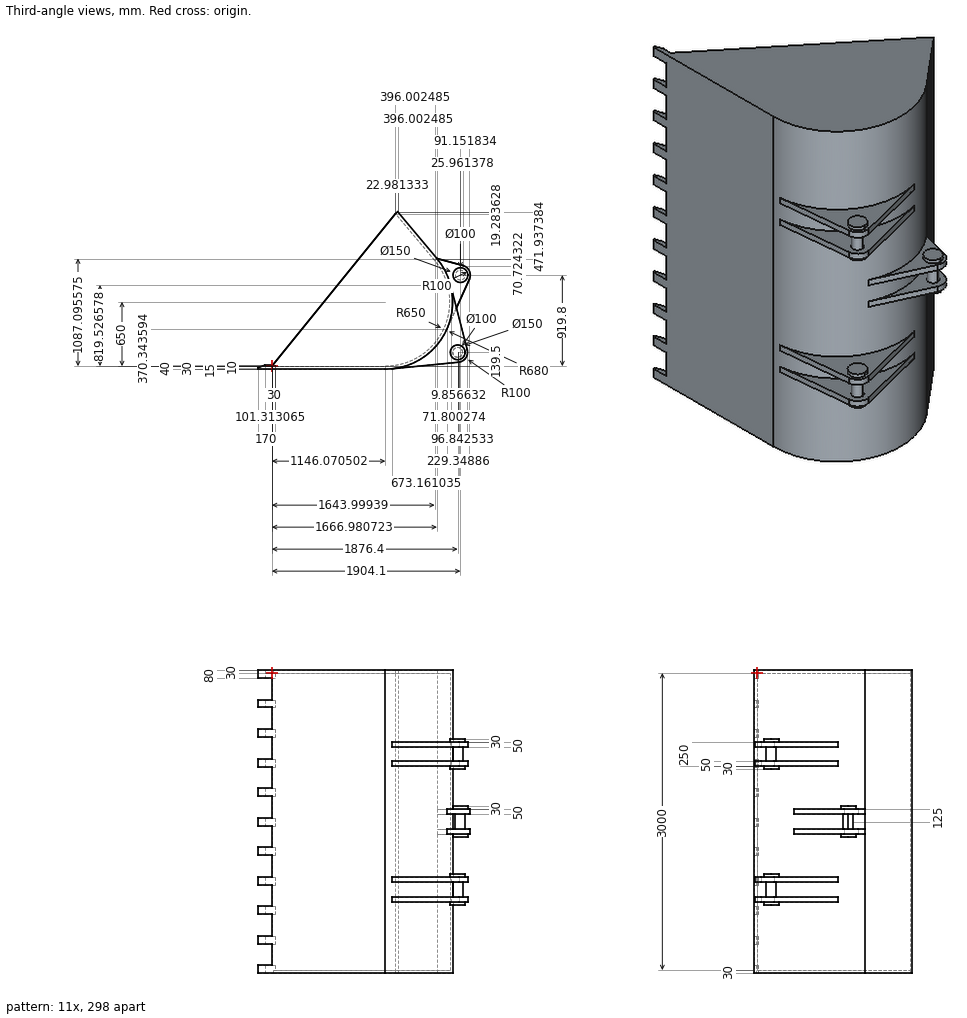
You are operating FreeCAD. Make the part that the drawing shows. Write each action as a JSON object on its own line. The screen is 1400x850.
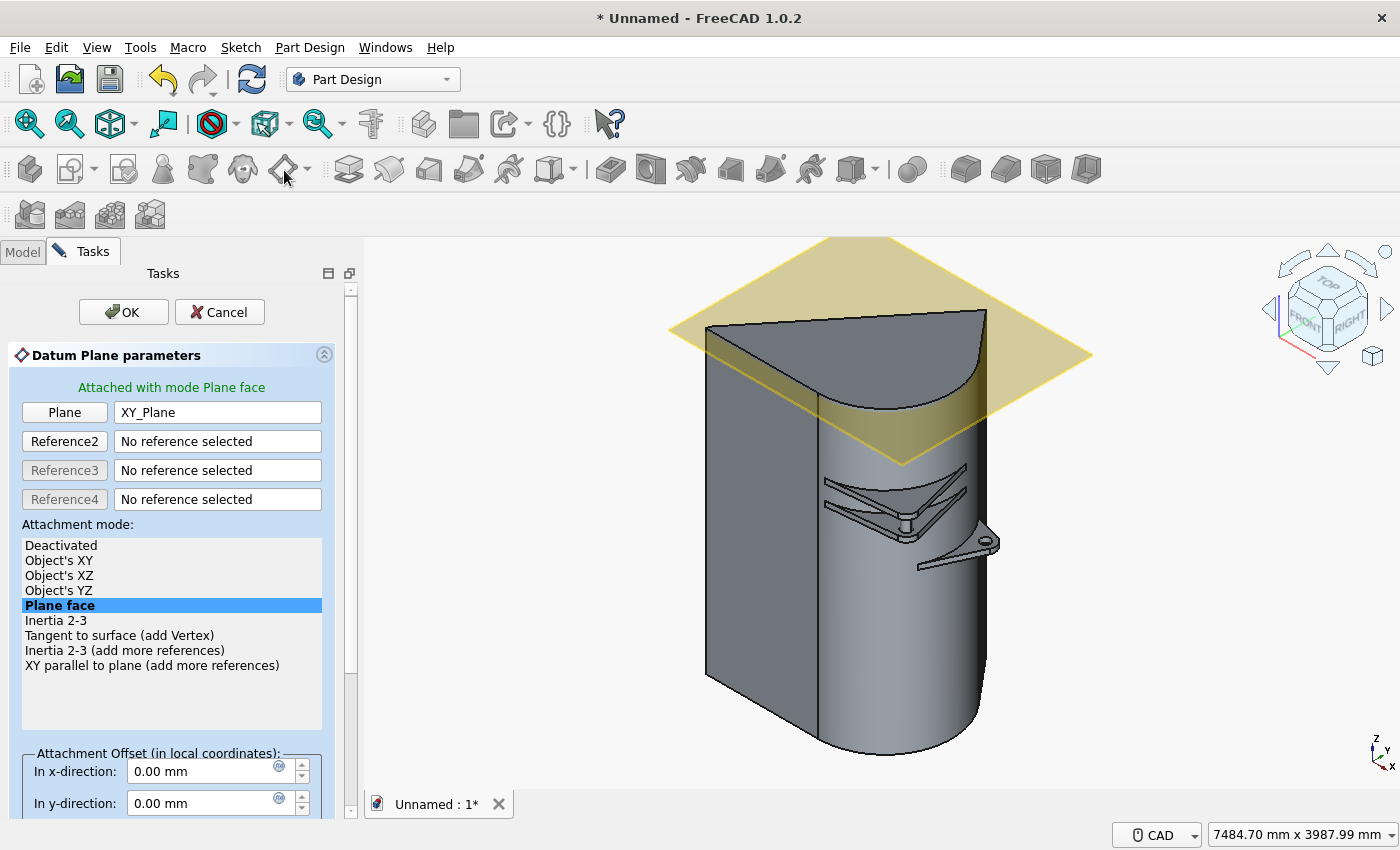
{"action": "scroll", "coordinate": [351, 550], "scroll_direction": "down", "scroll_amount": 2}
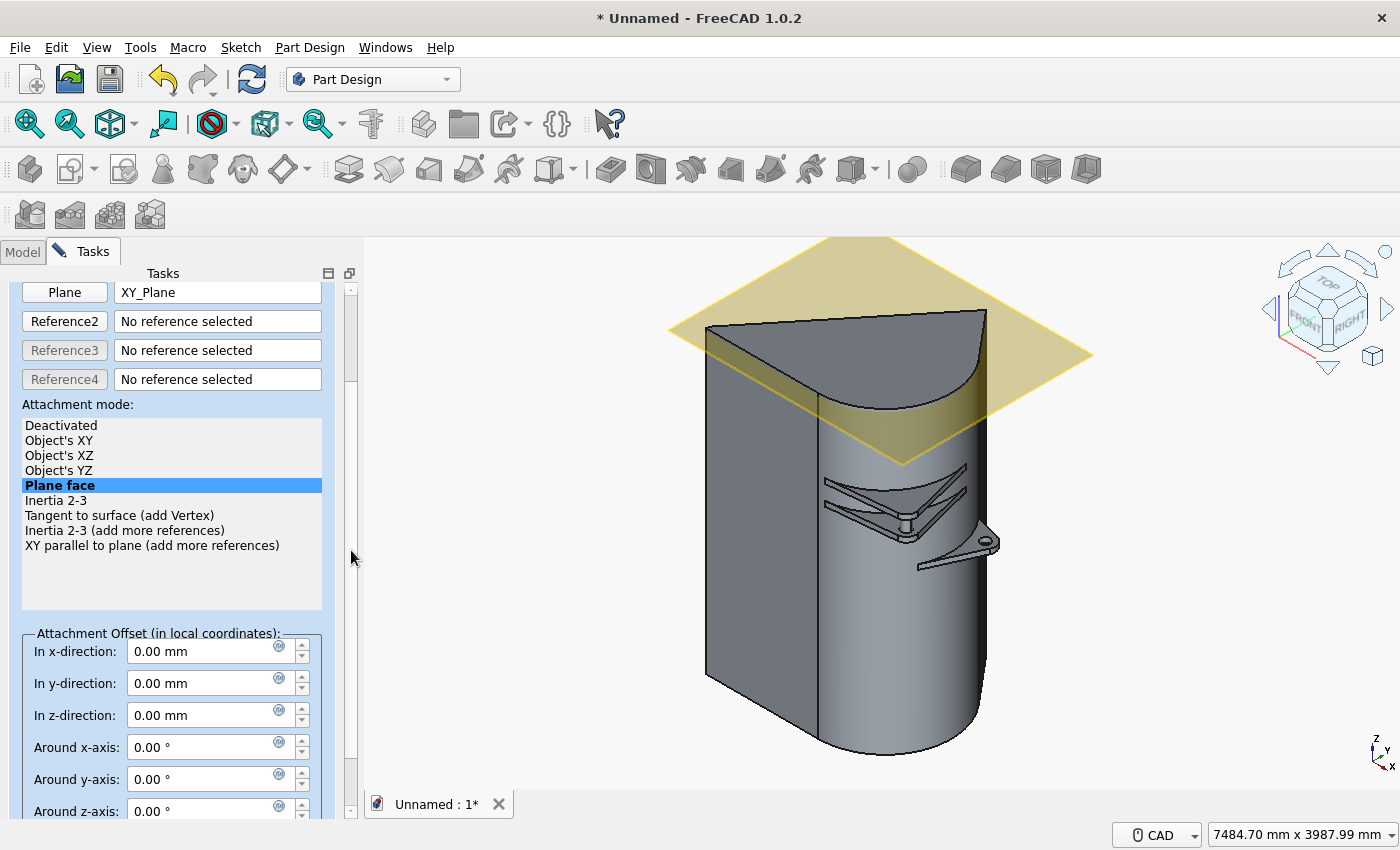
{"action": "triple_click", "coordinate": [210, 715]}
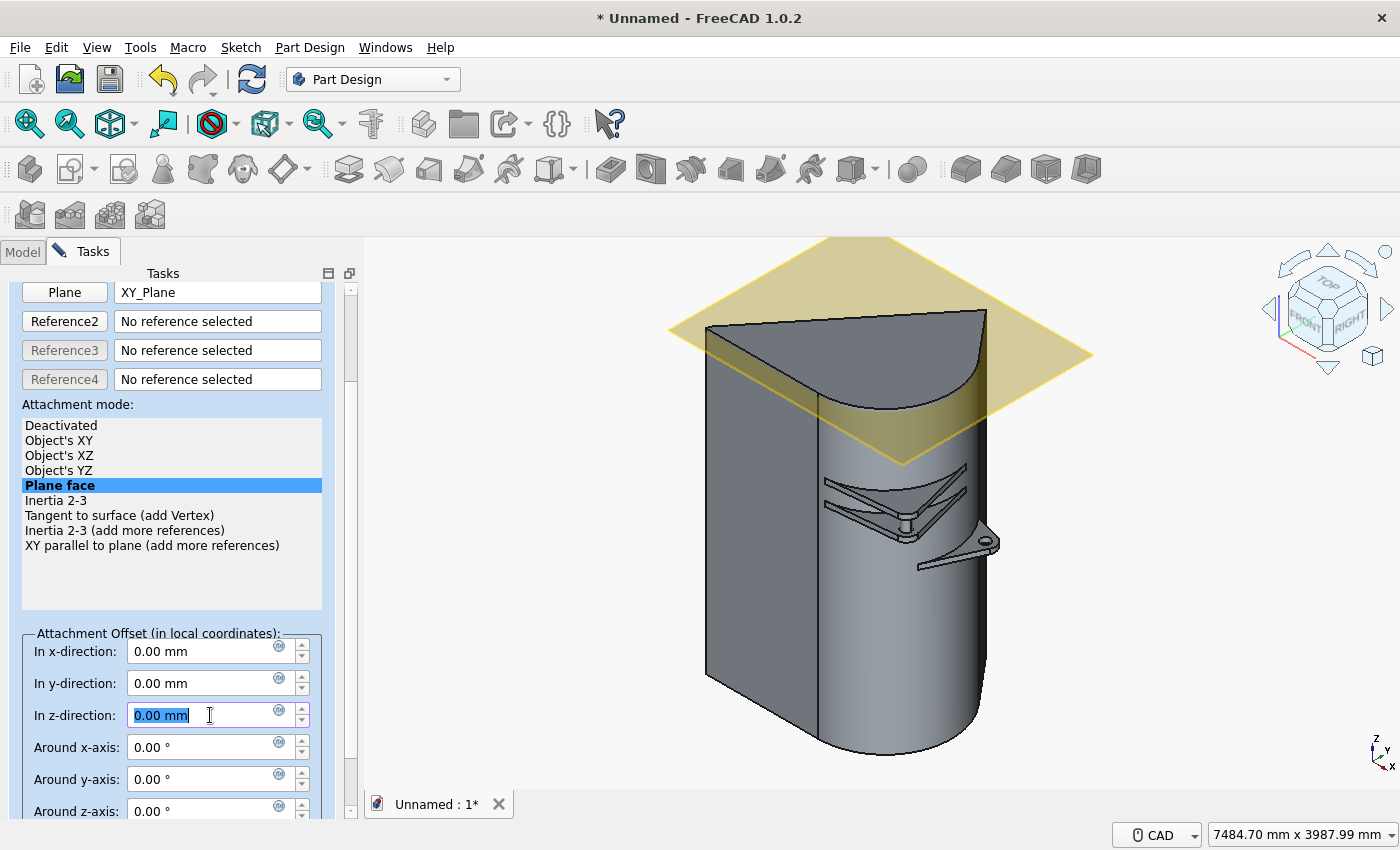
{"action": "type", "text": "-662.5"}
{"action": "key", "text": "Tab"}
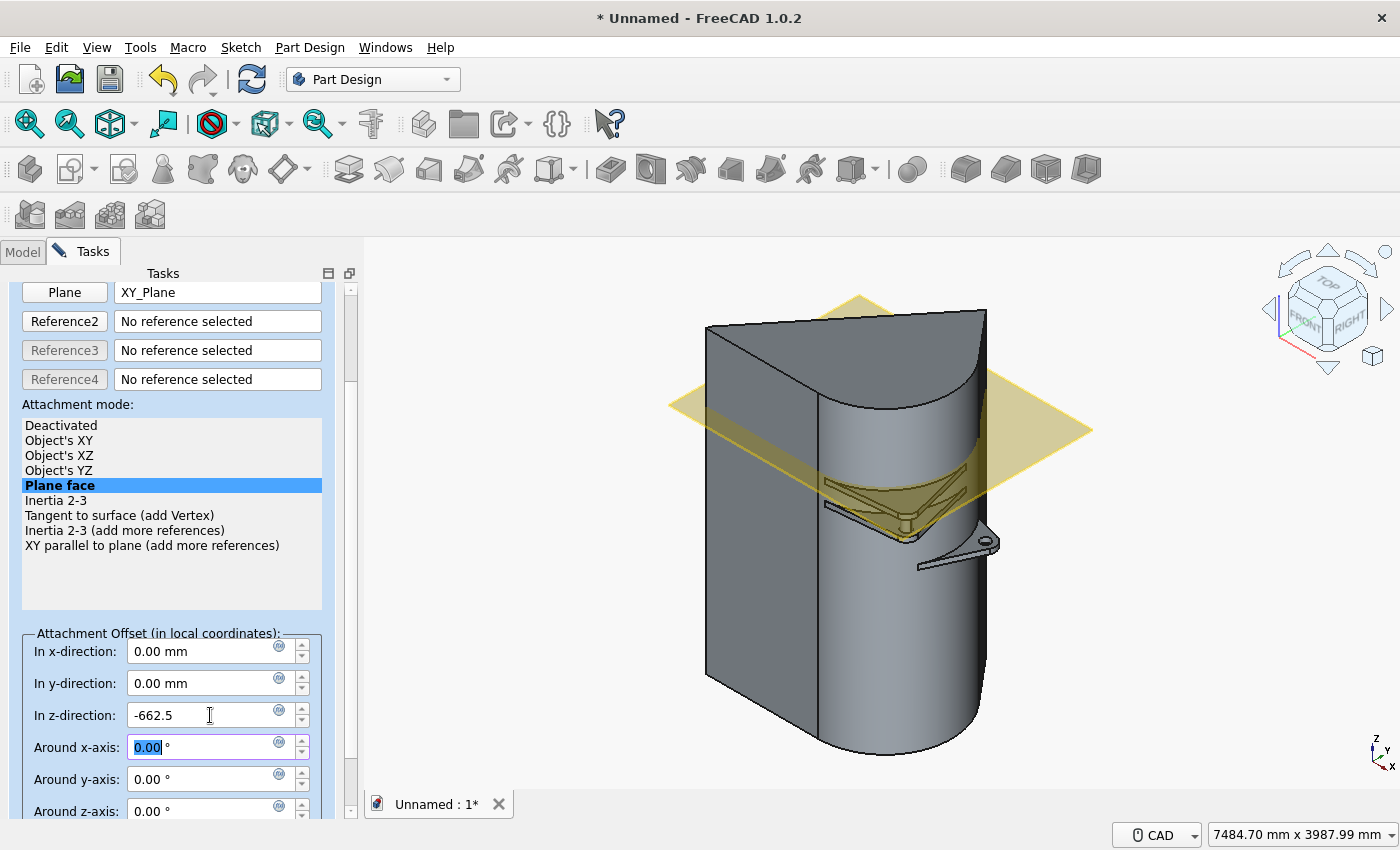
{"action": "scroll", "coordinate": [351, 550], "scroll_direction": "up", "scroll_amount": 3}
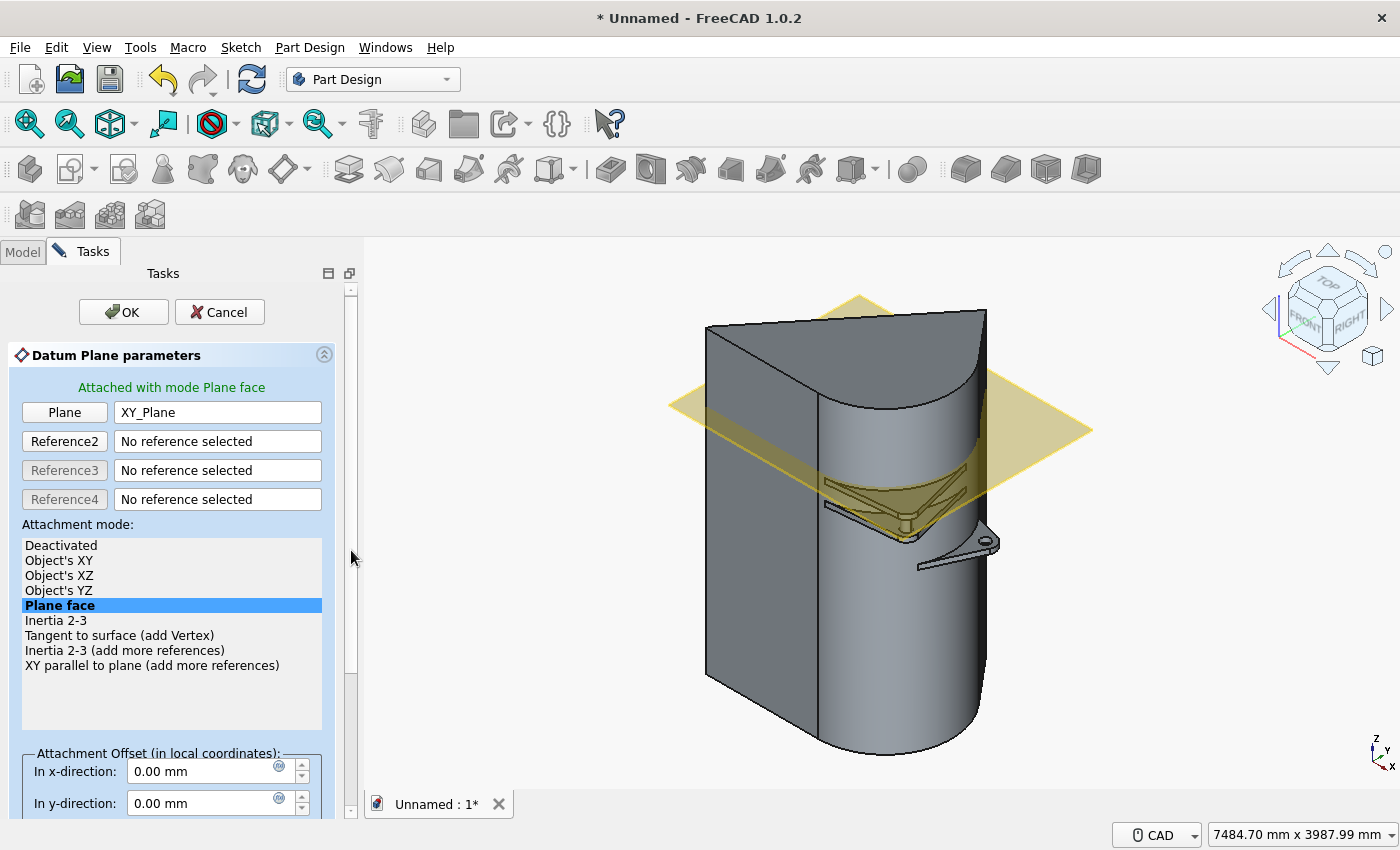
{"action": "left_click", "coordinate": [124, 312]}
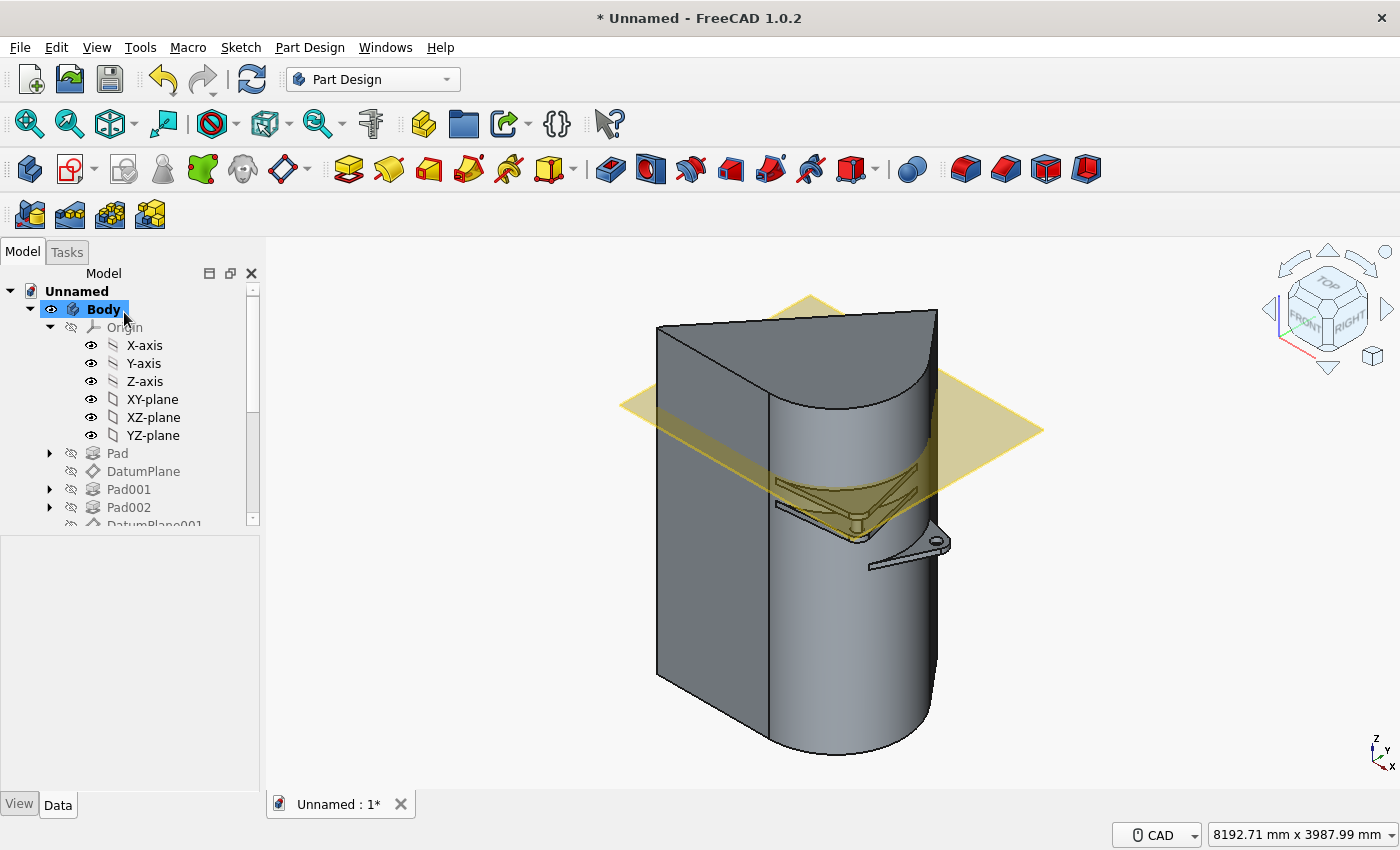
{"action": "scroll", "coordinate": [100, 413], "scroll_direction": "down", "scroll_amount": 3}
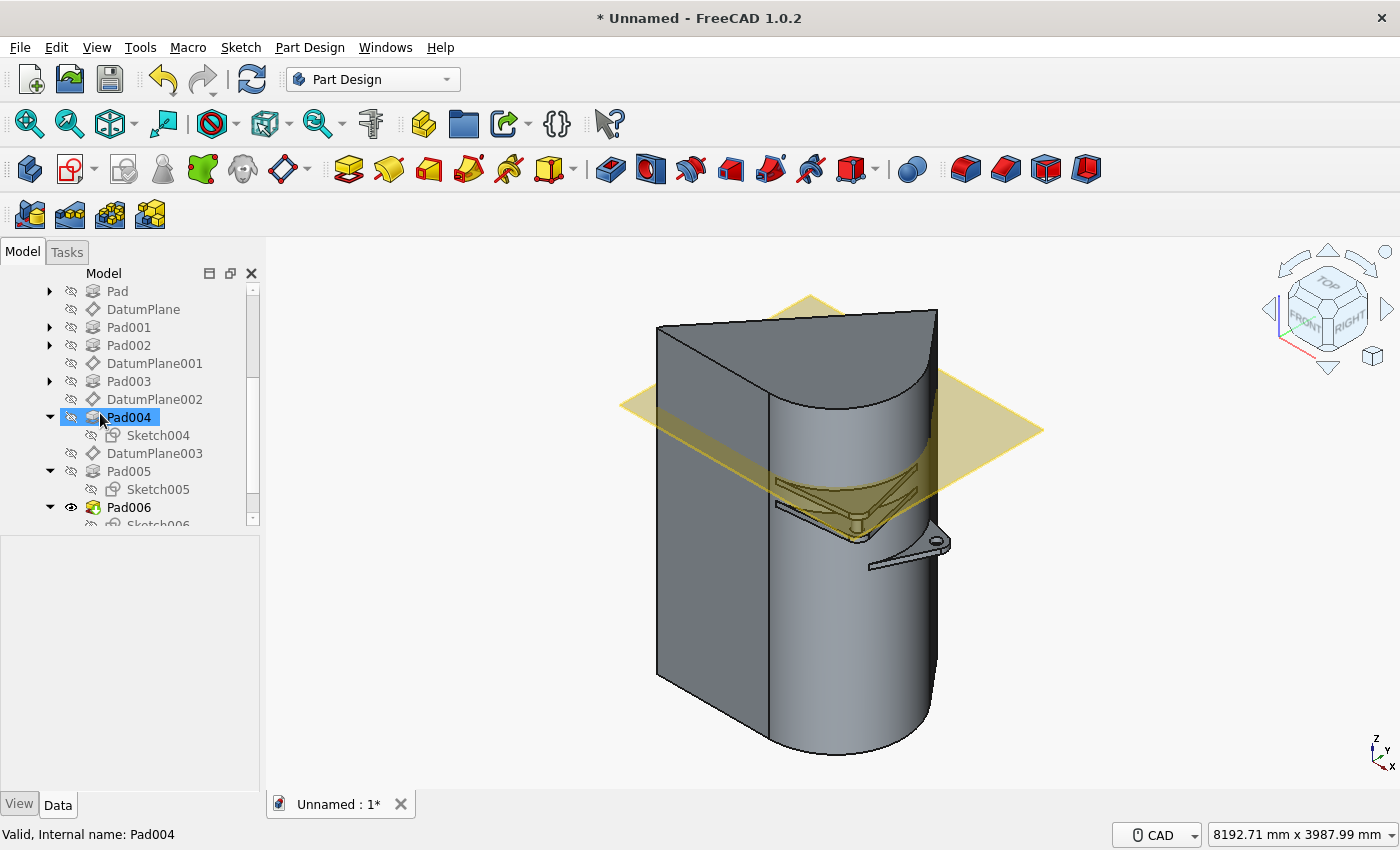
{"action": "scroll", "coordinate": [140, 413], "scroll_direction": "up", "scroll_amount": 15}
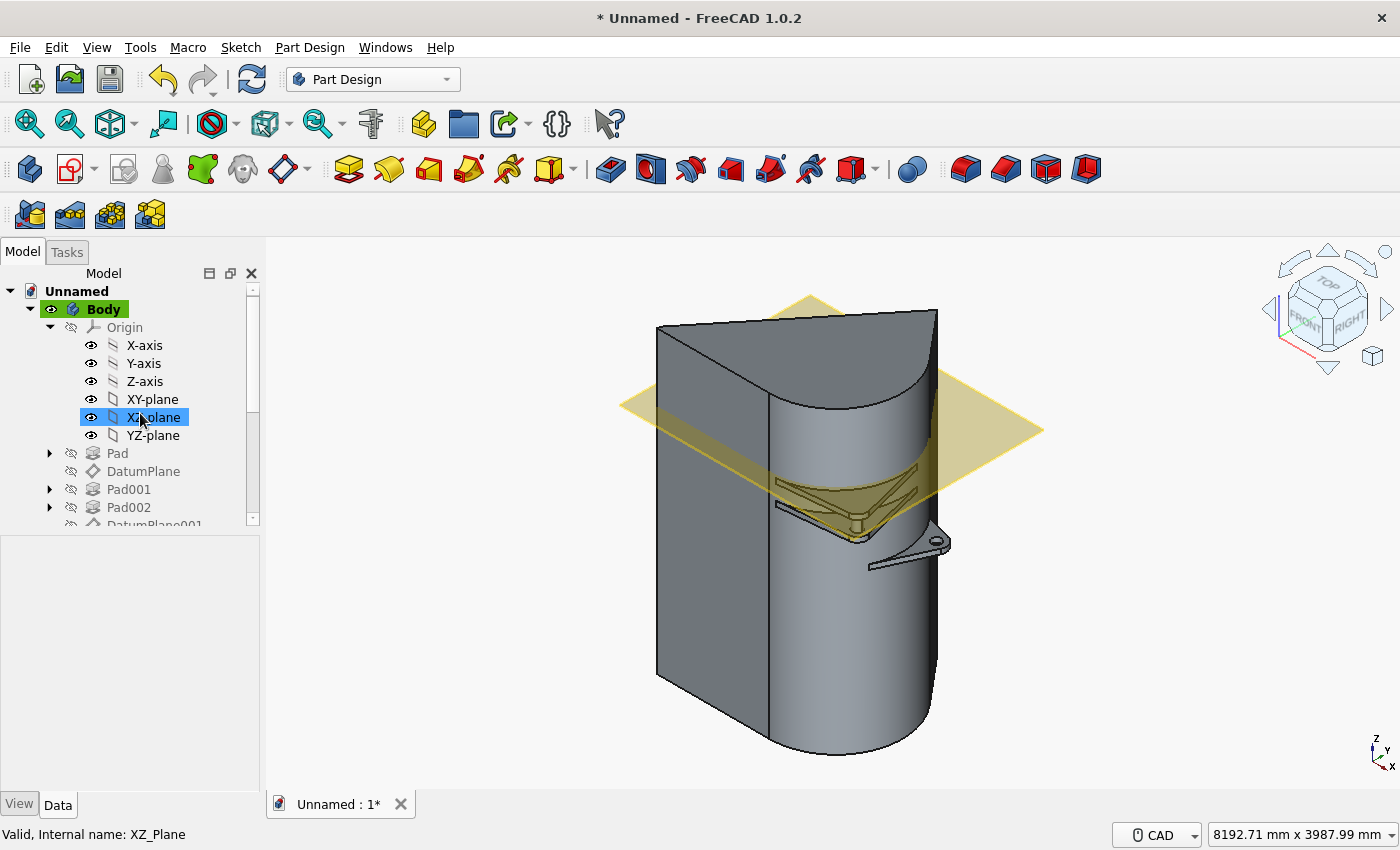
{"action": "scroll", "coordinate": [100, 413], "scroll_direction": "down", "scroll_amount": 6}